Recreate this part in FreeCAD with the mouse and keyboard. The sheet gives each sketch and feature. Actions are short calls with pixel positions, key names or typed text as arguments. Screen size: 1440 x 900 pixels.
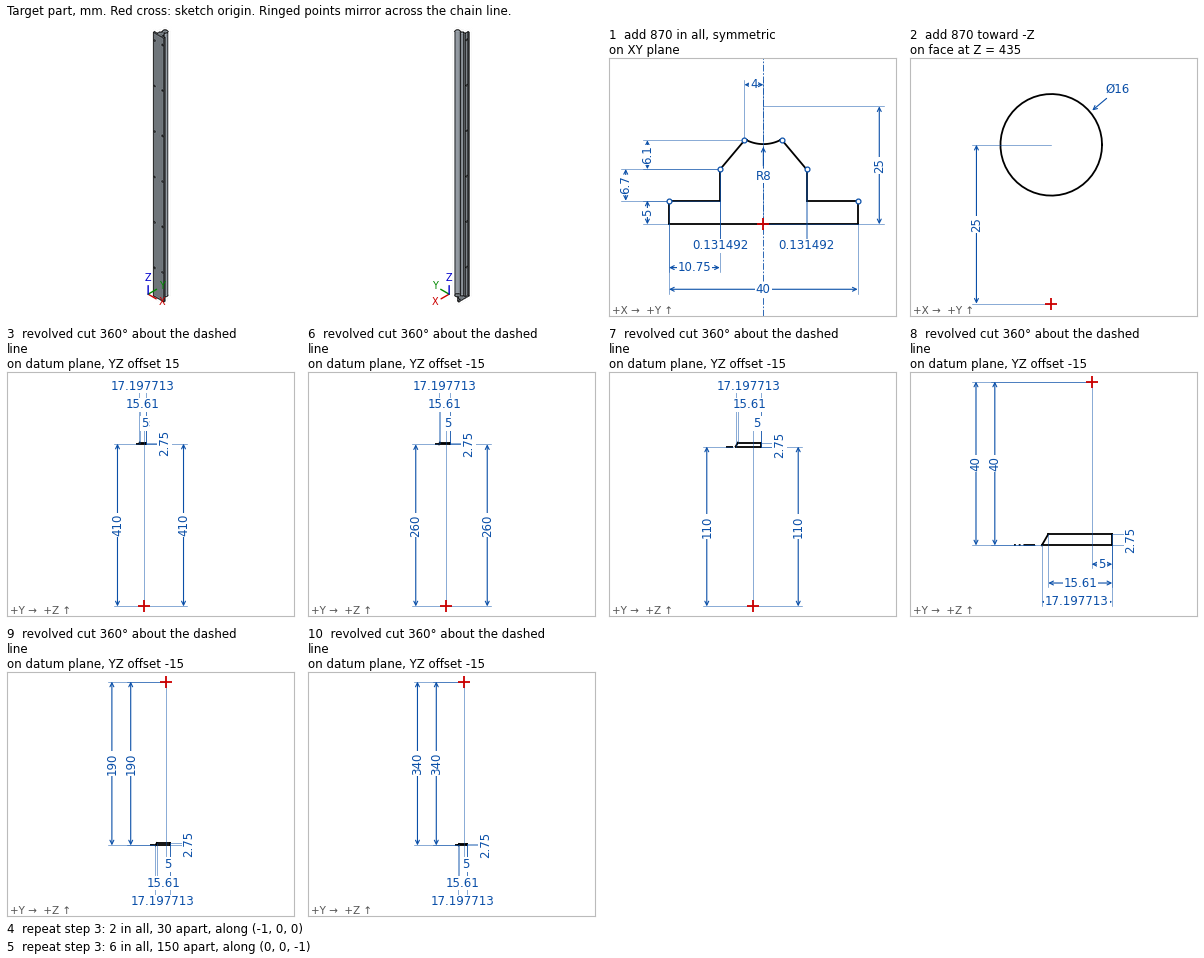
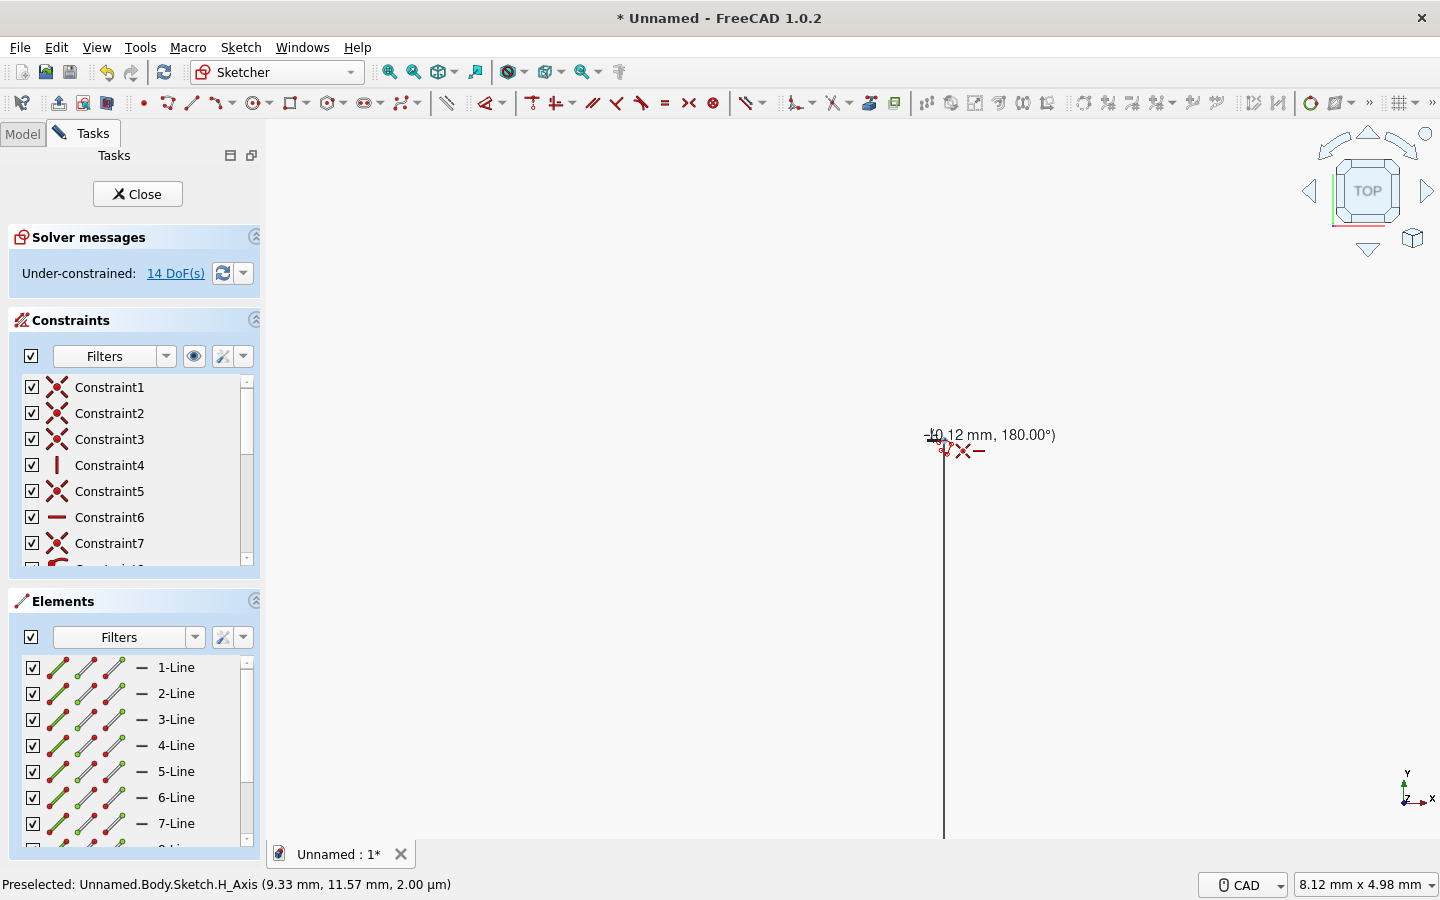
click(923, 431)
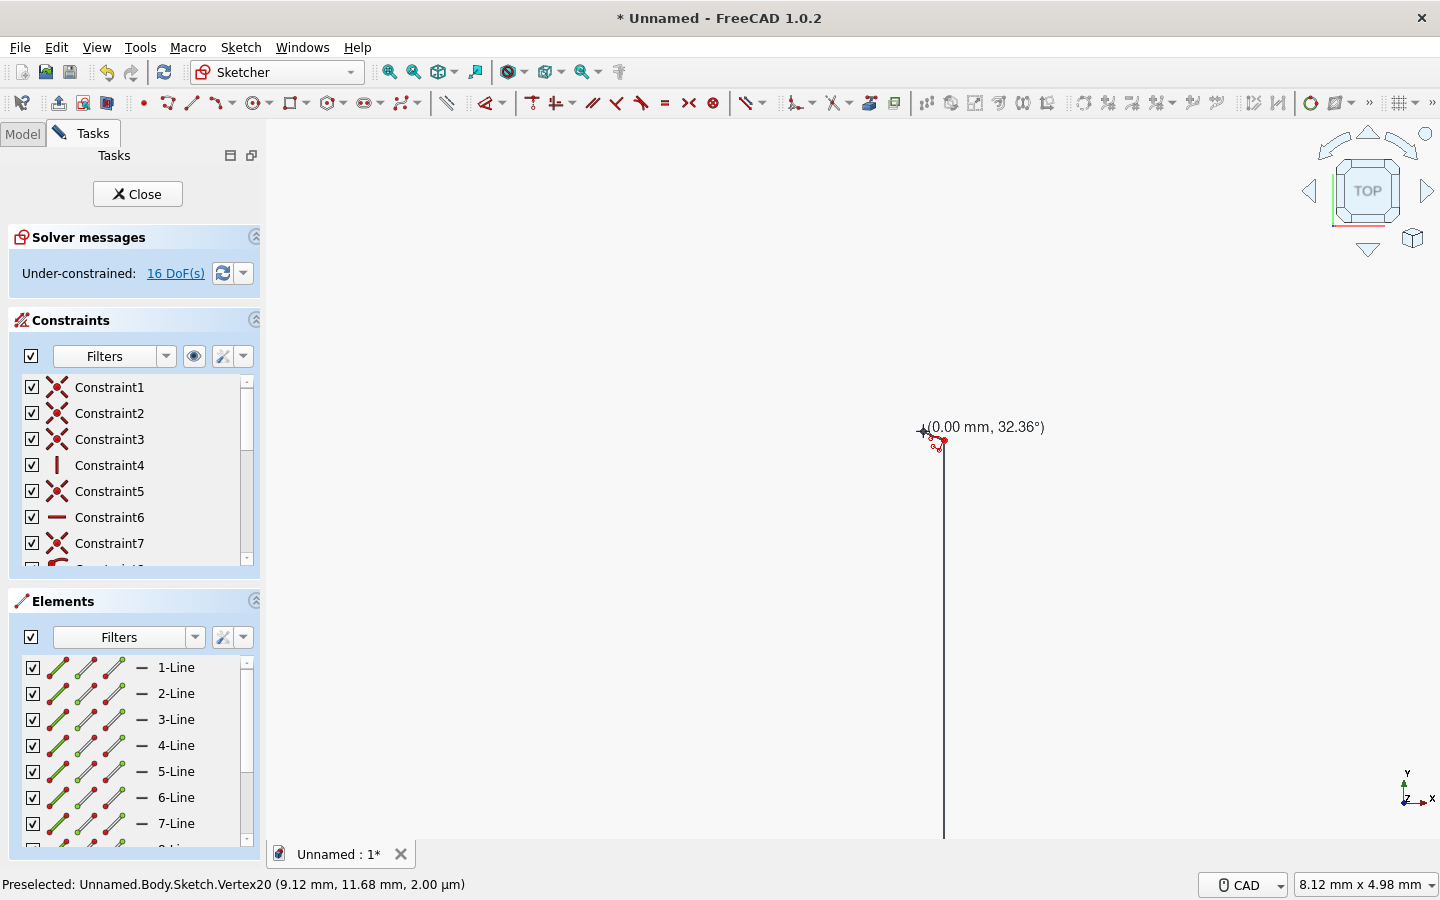
scroll(932, 435, down, 11)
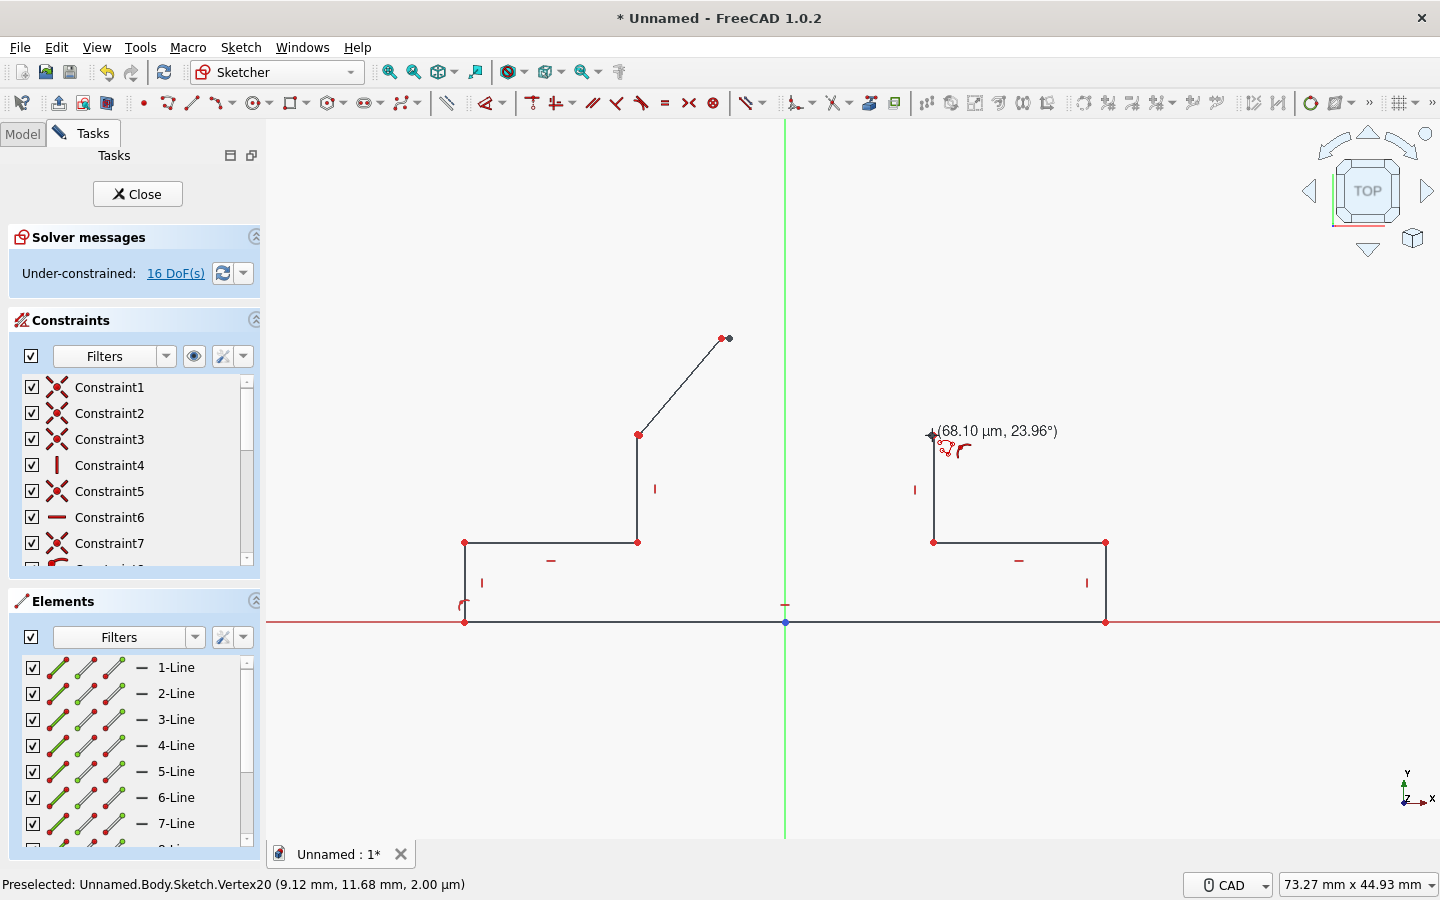
click(850, 337)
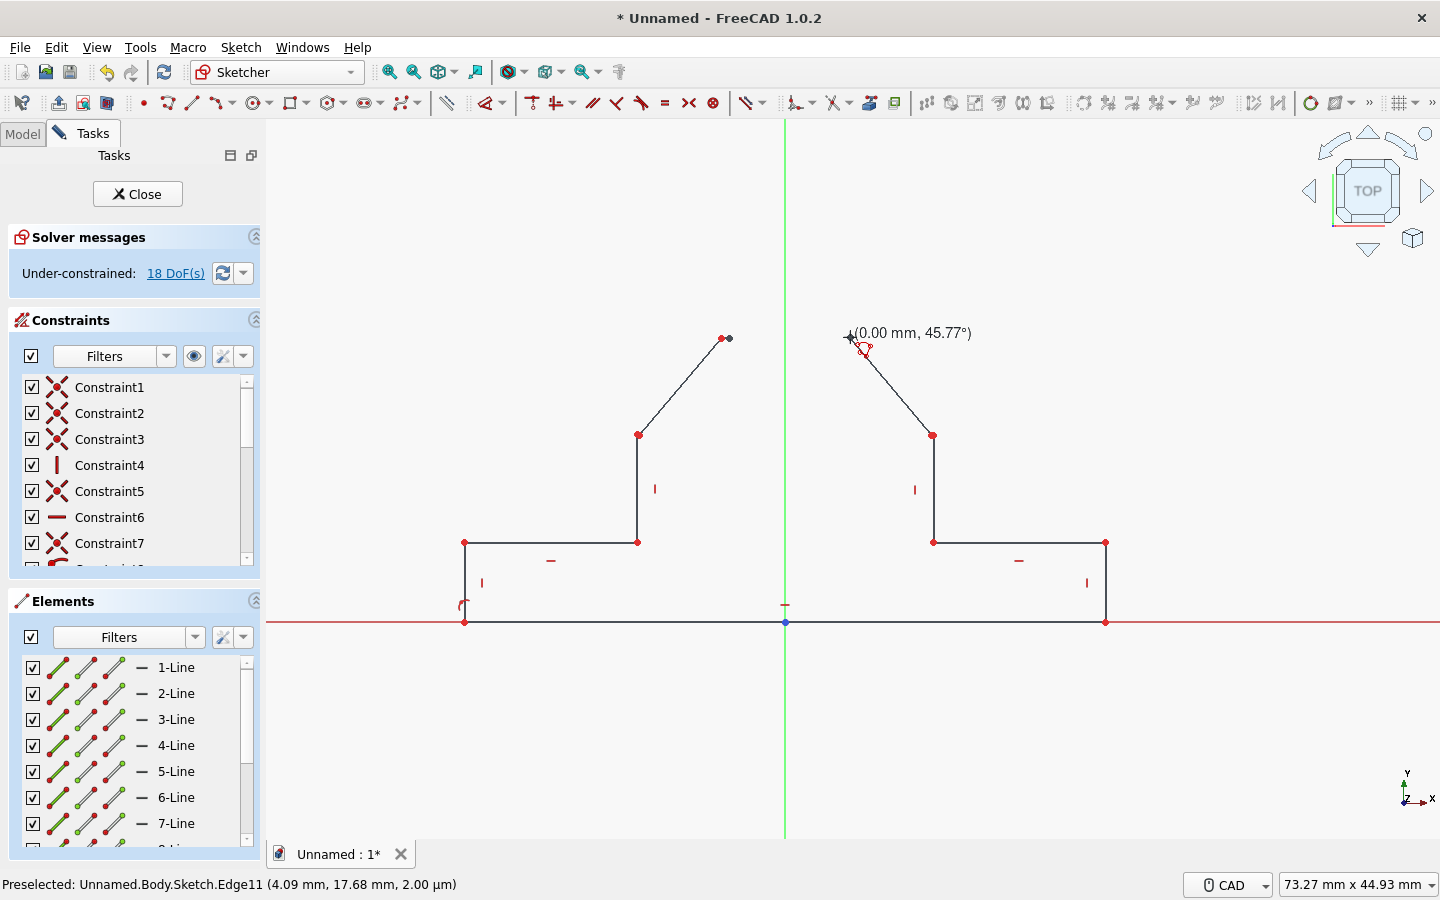
scroll(841, 337, up, 4)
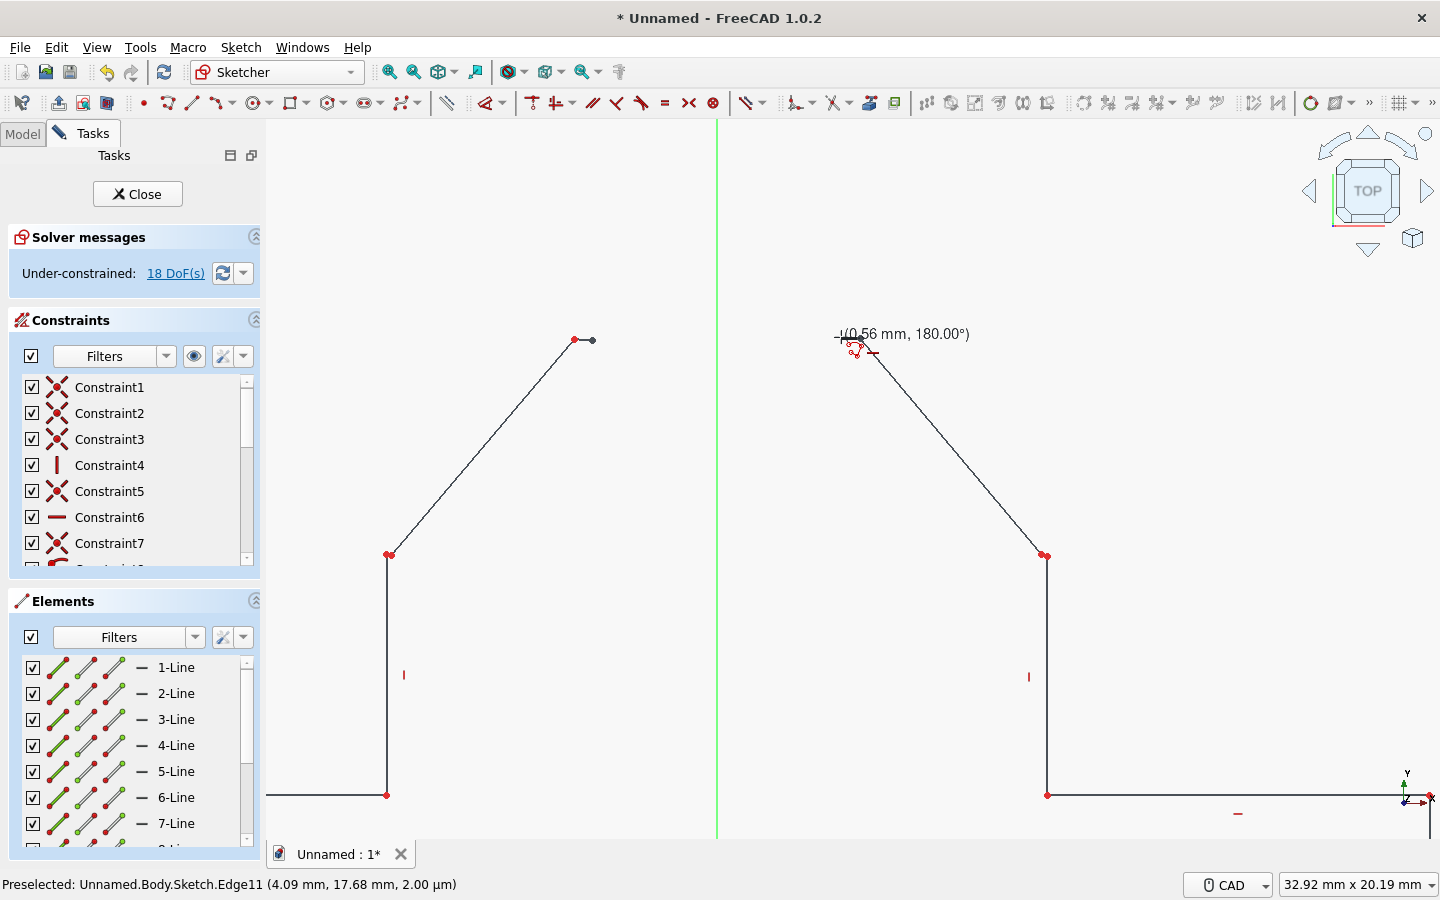
click(841, 337)
right_click(841, 337)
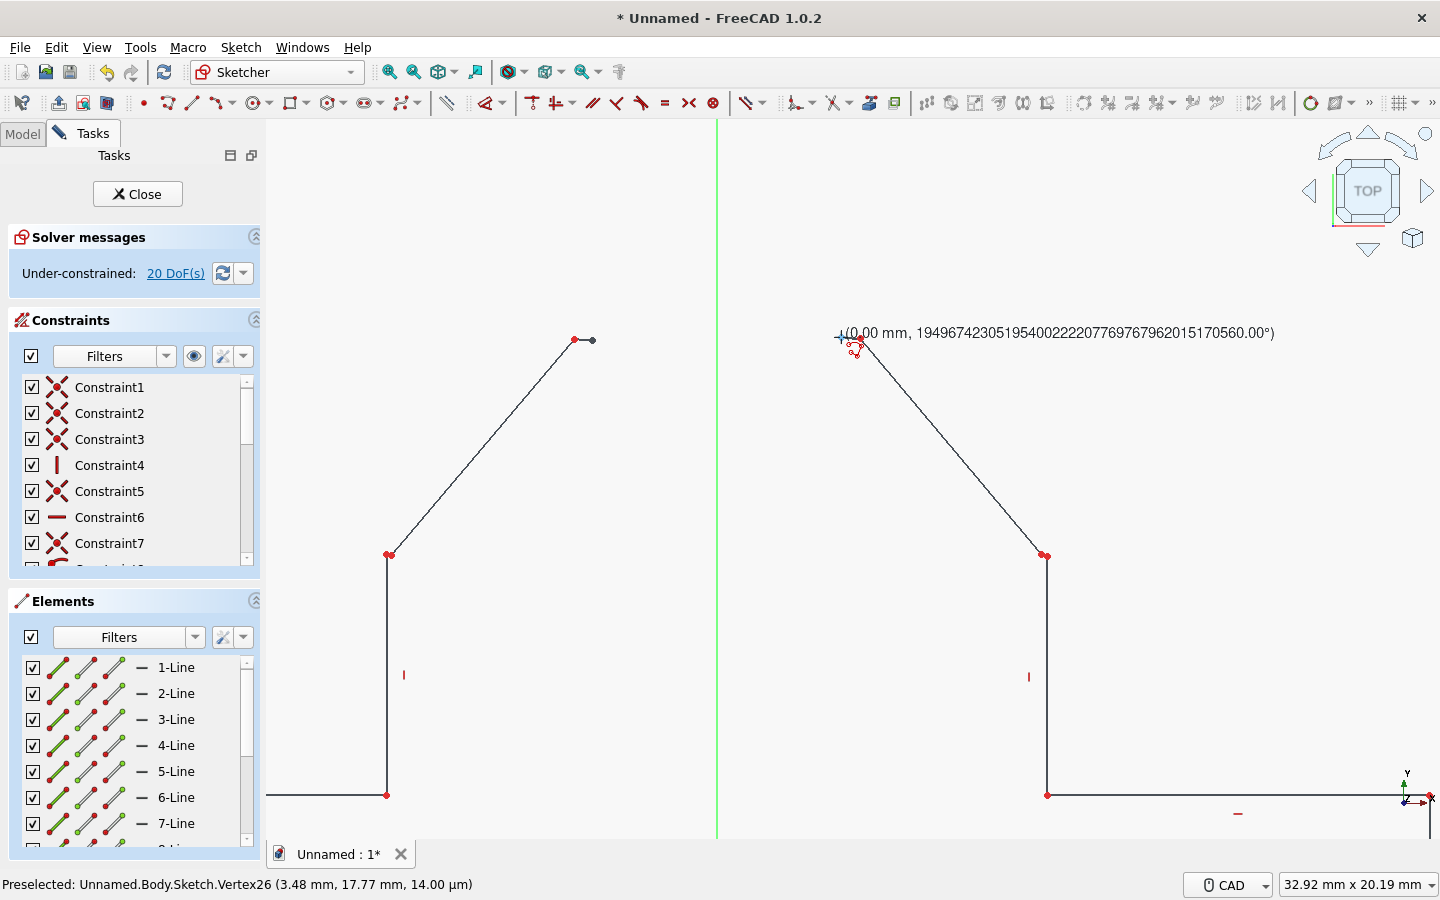
click(216, 104)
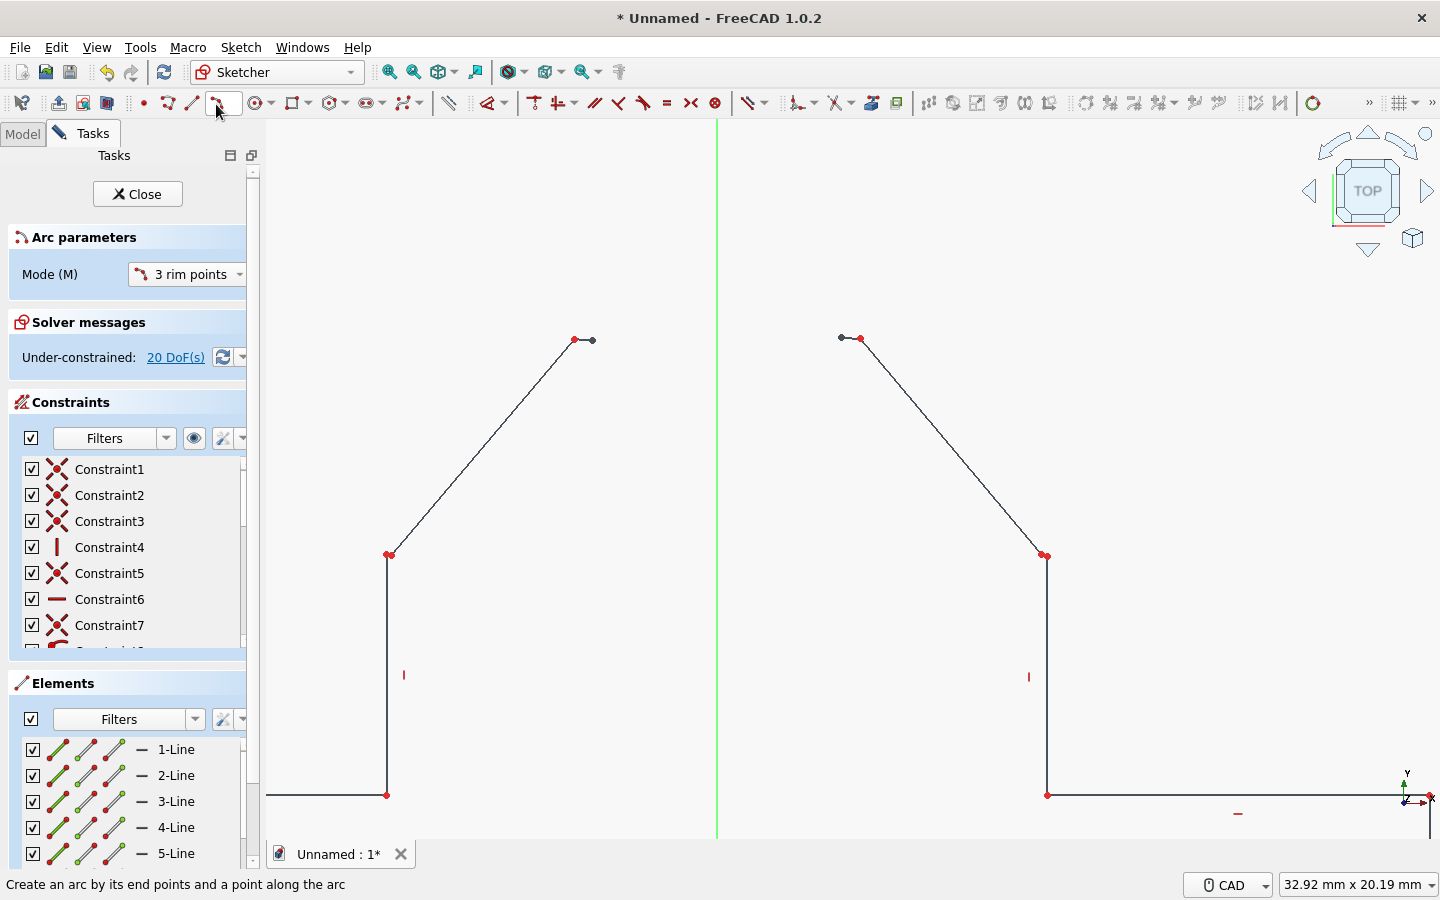
scroll(841, 337, up, 3)